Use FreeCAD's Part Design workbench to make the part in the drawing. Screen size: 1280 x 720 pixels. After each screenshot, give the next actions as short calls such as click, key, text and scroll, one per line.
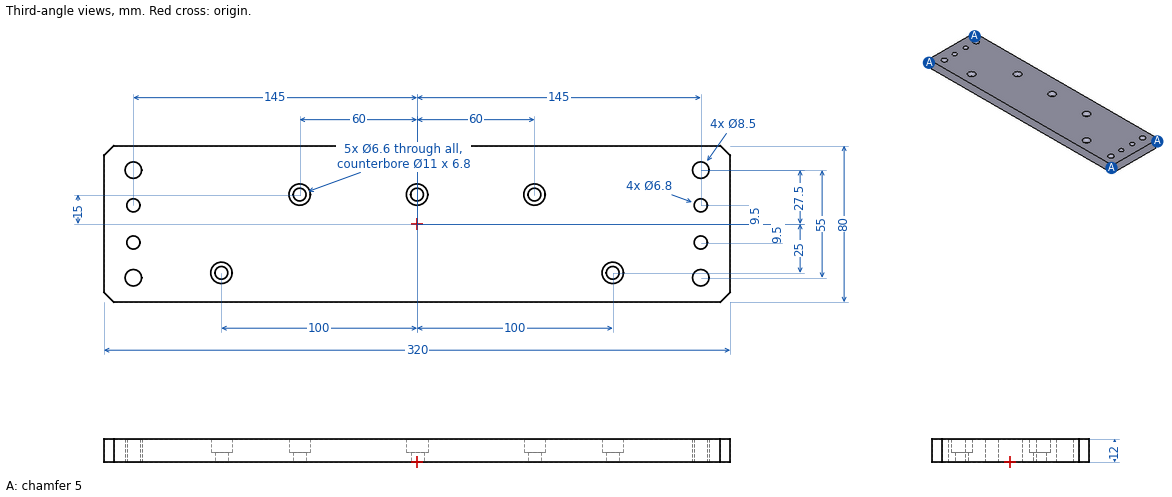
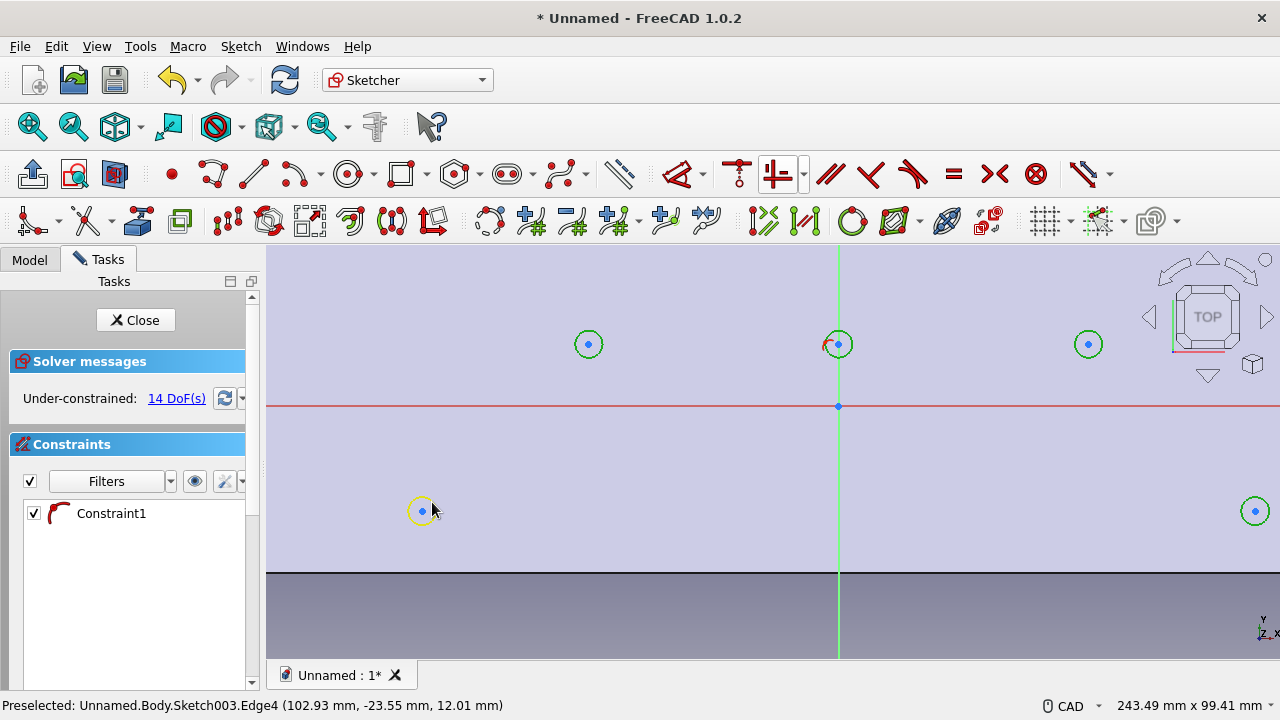
click(432, 501)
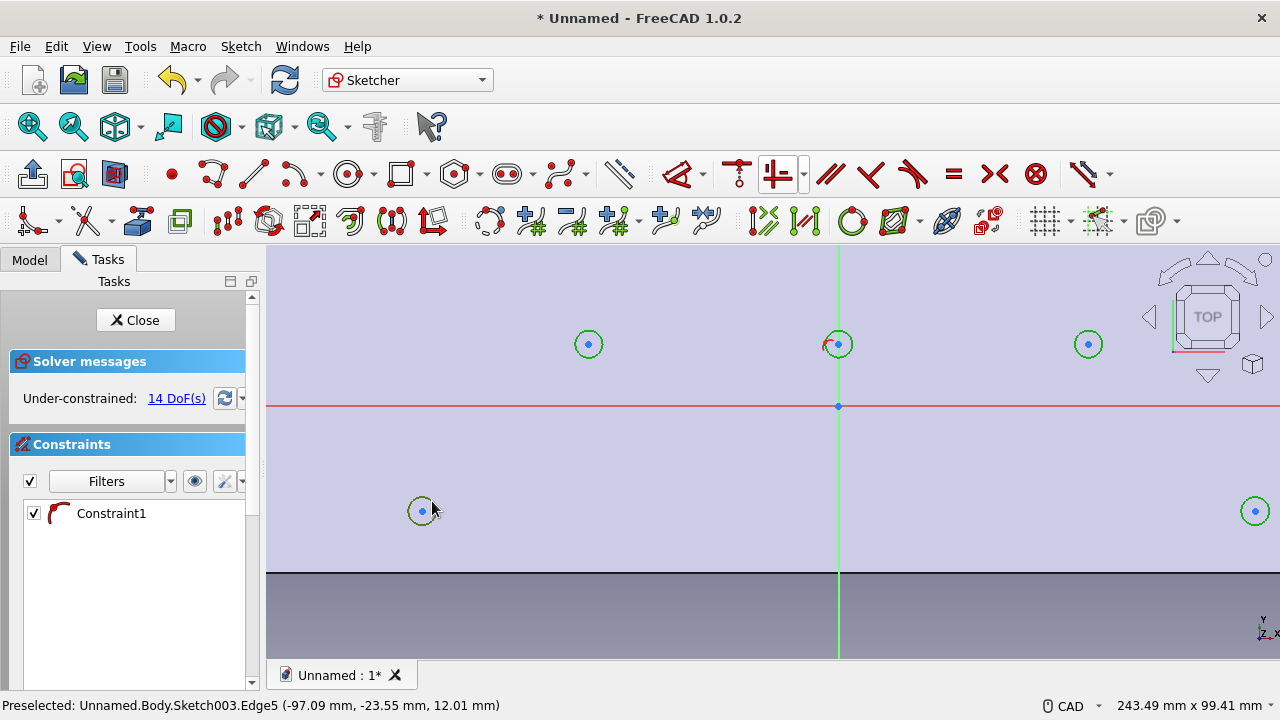
click(954, 174)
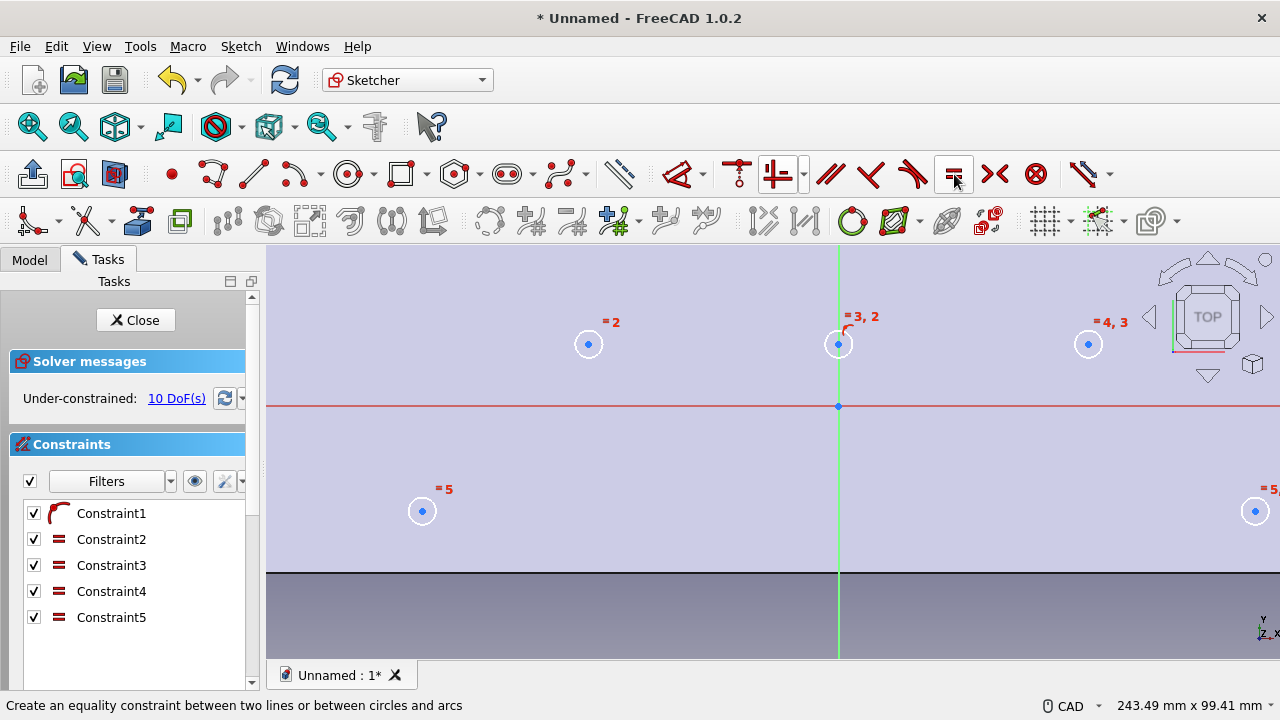
click(676, 174)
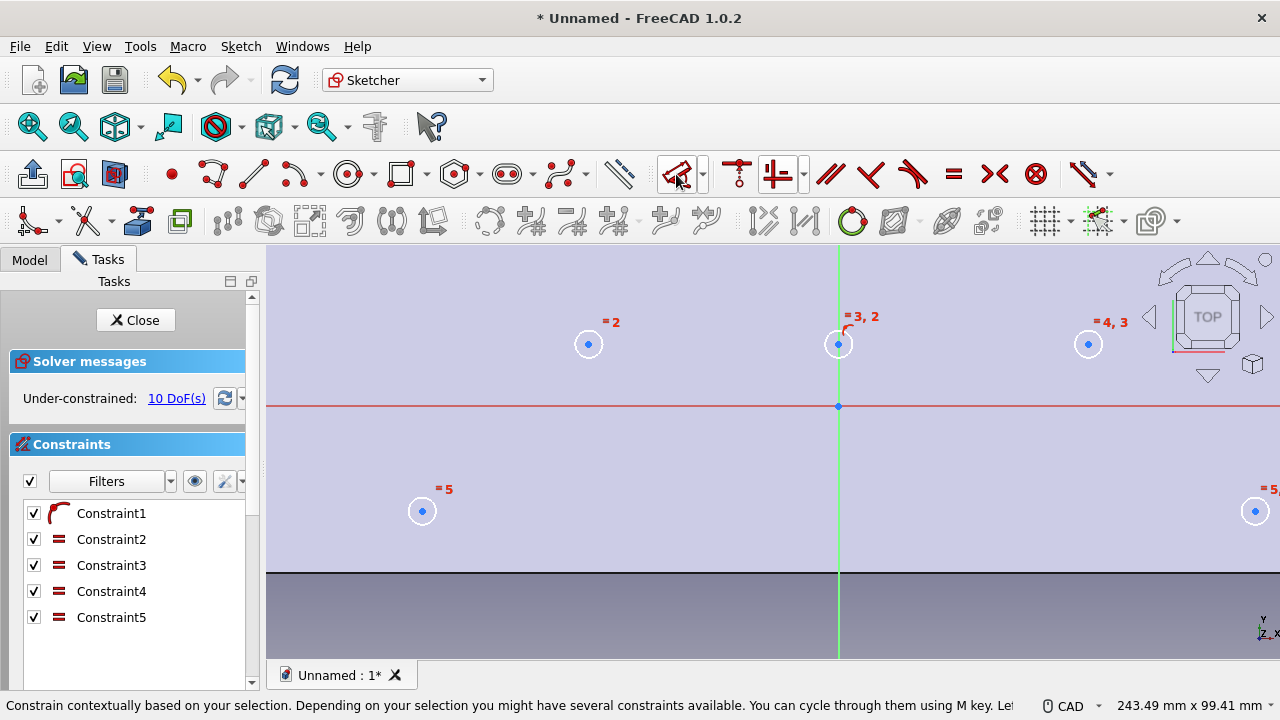
scroll(599, 335, up, 2)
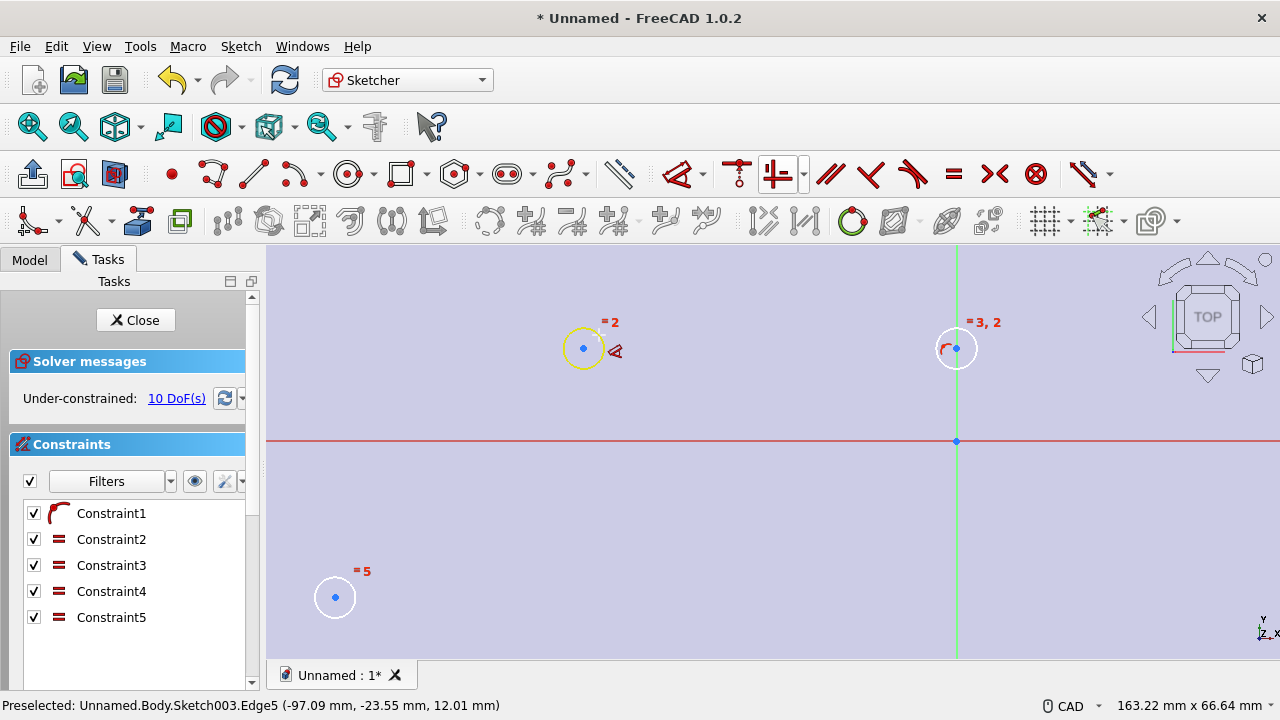
click(598, 334)
click(620, 311)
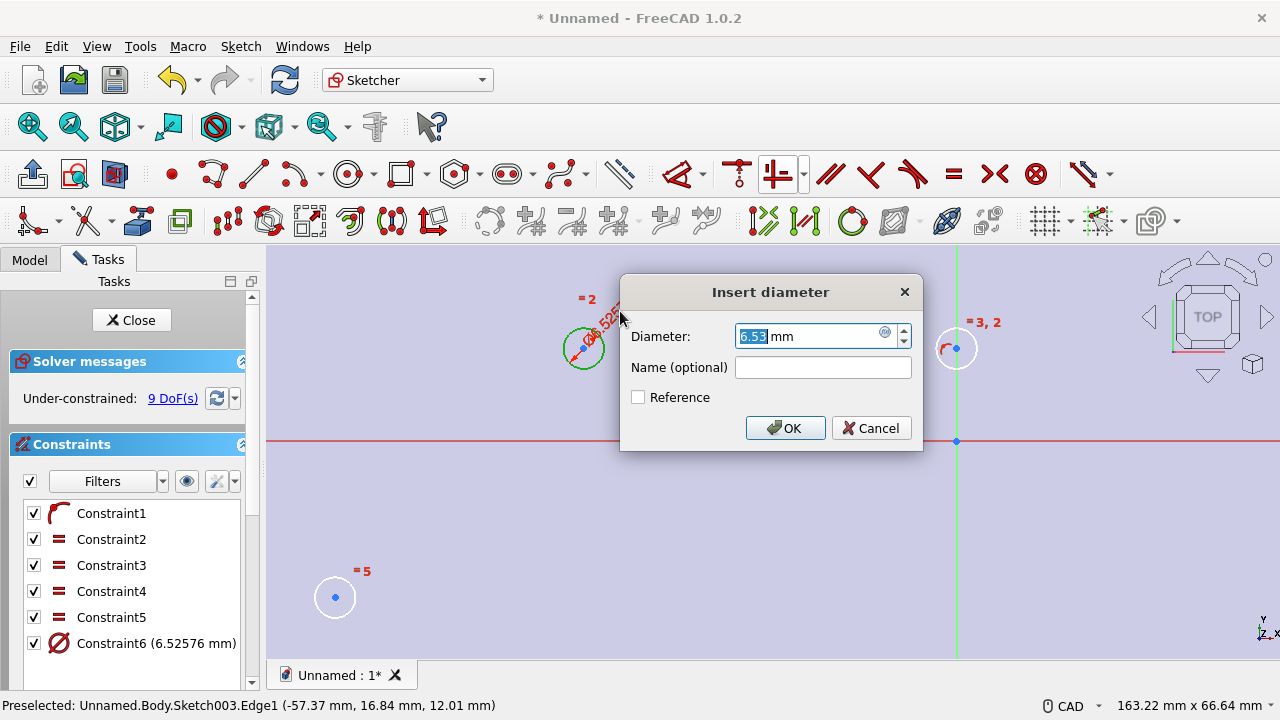
text(6.6)
key(Return)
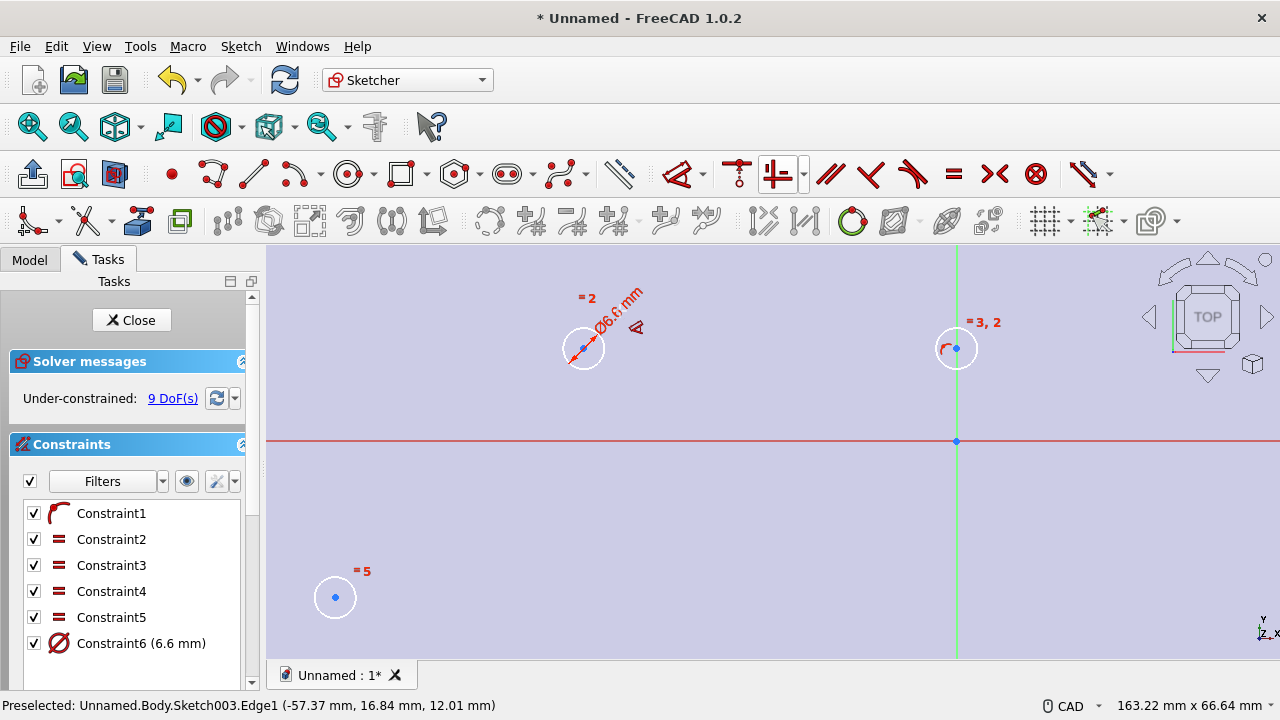
click(584, 349)
click(770, 315)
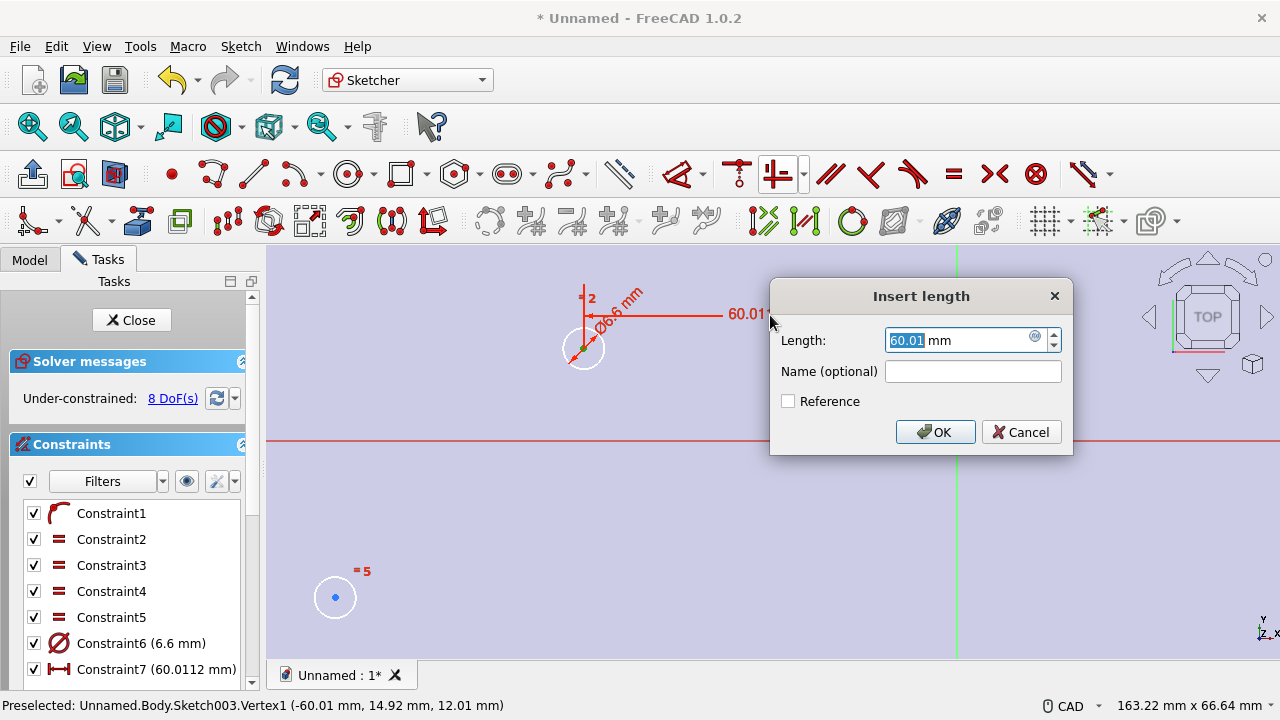
text(60)
key(Return)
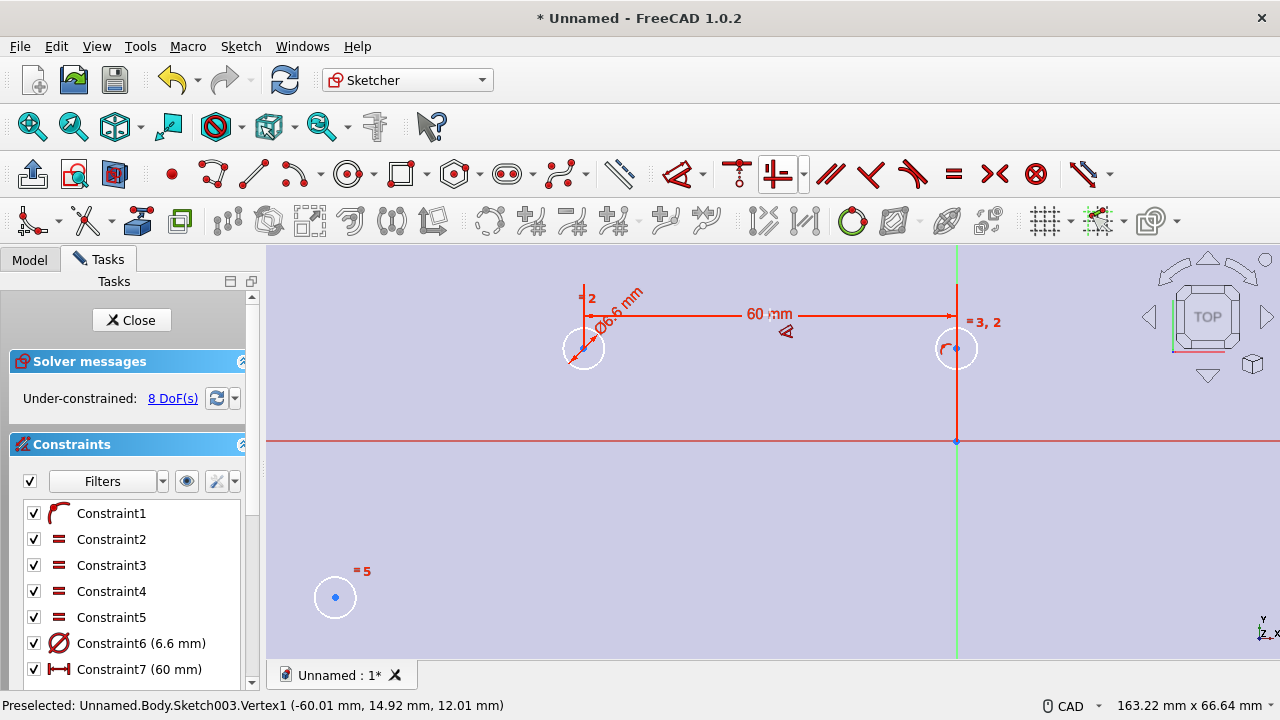
click(584, 349)
click(550, 395)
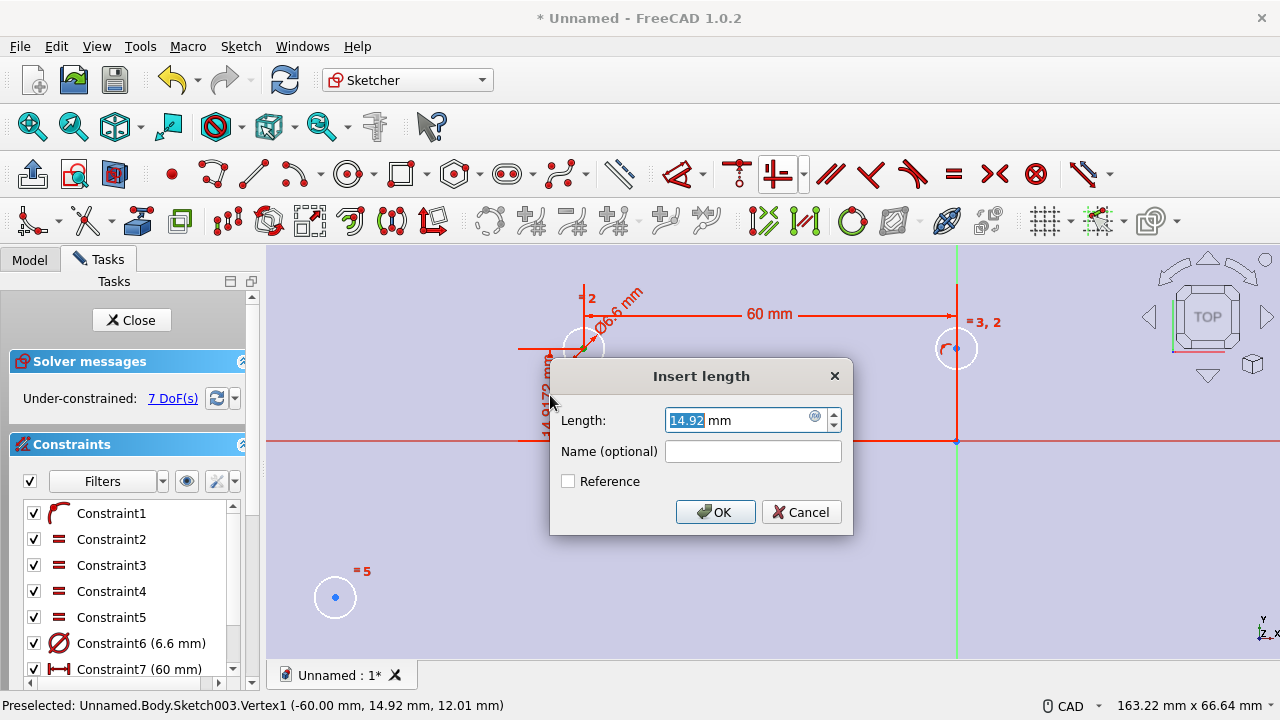
text(15)
key(Return)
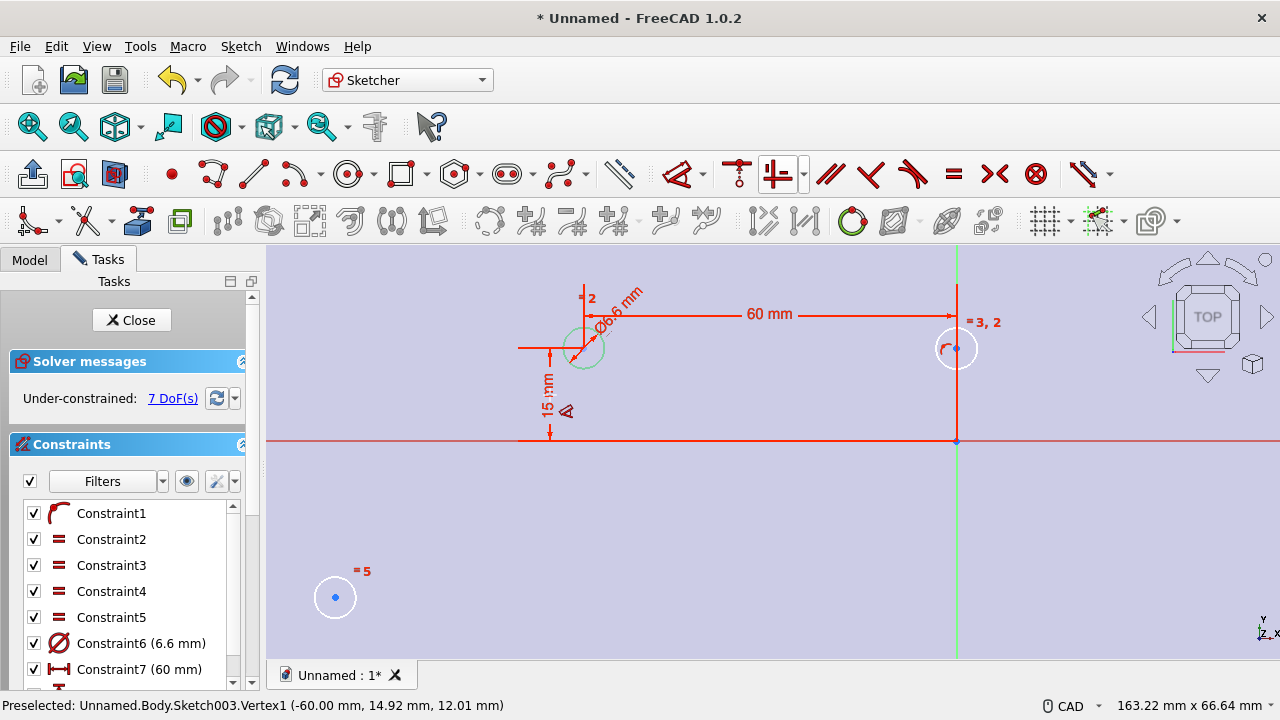
click(957, 349)
click(991, 395)